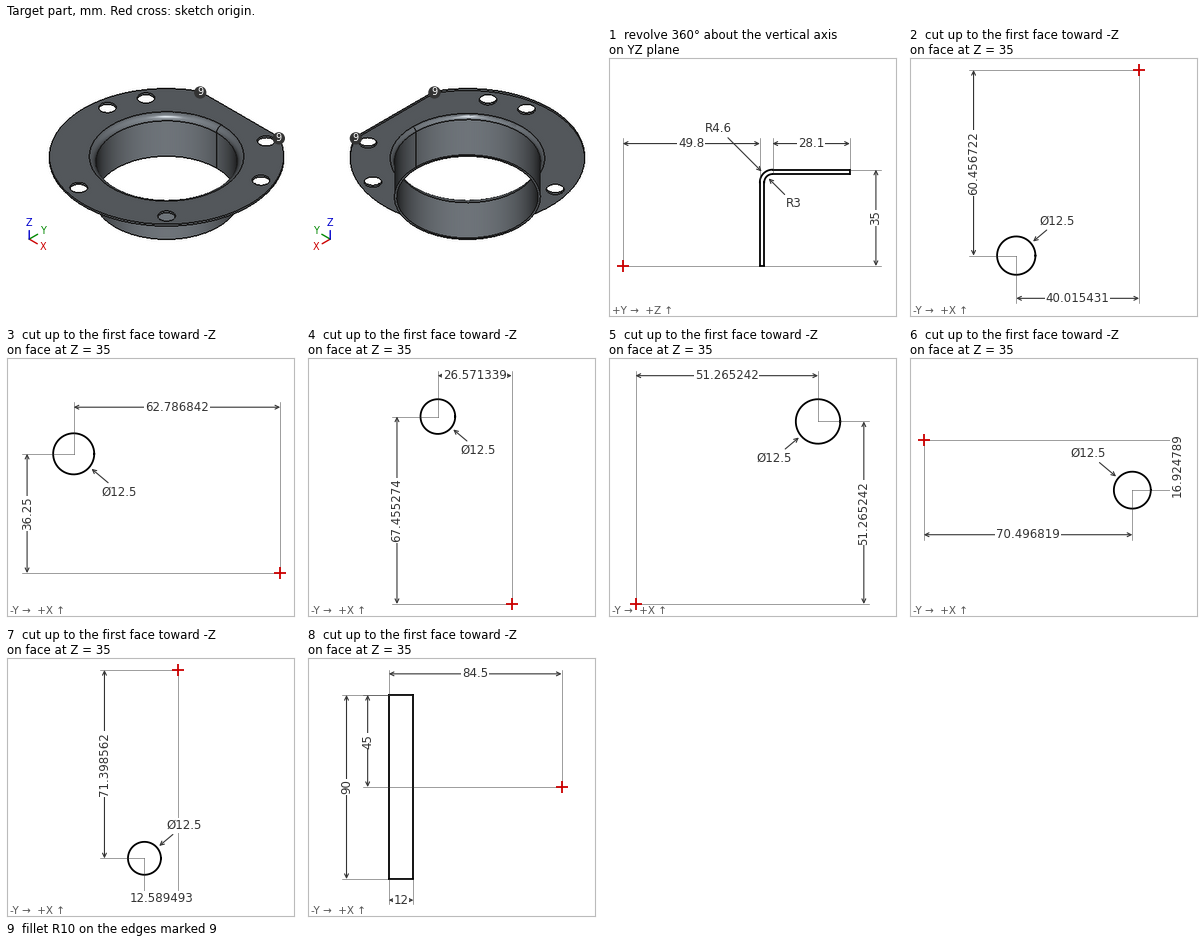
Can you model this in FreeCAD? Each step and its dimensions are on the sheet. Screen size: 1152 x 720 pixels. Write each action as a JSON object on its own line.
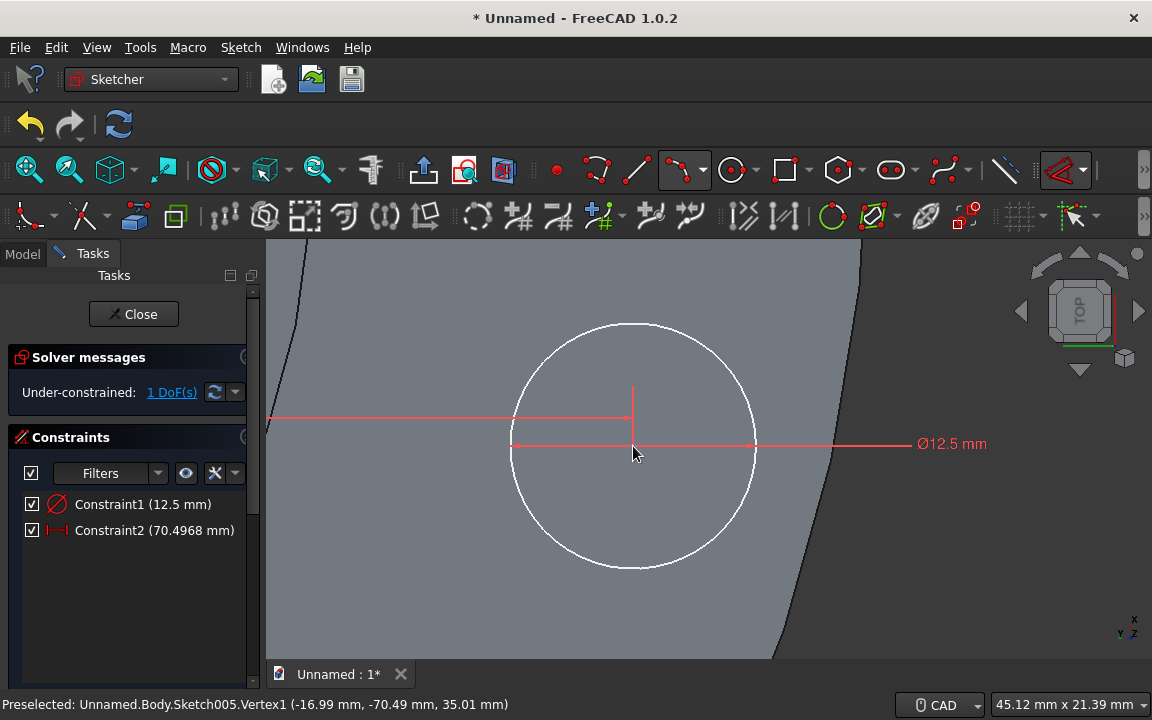
{"action": "left_click", "coordinate": [633, 446]}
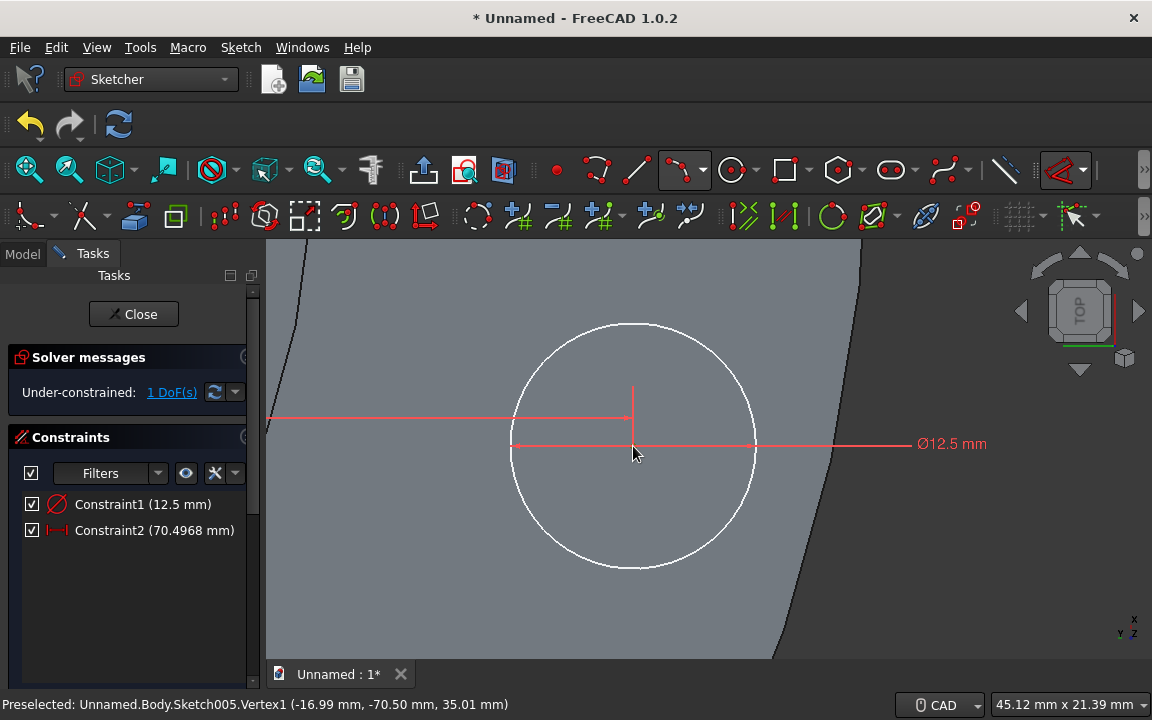
{"action": "key", "text": "i"}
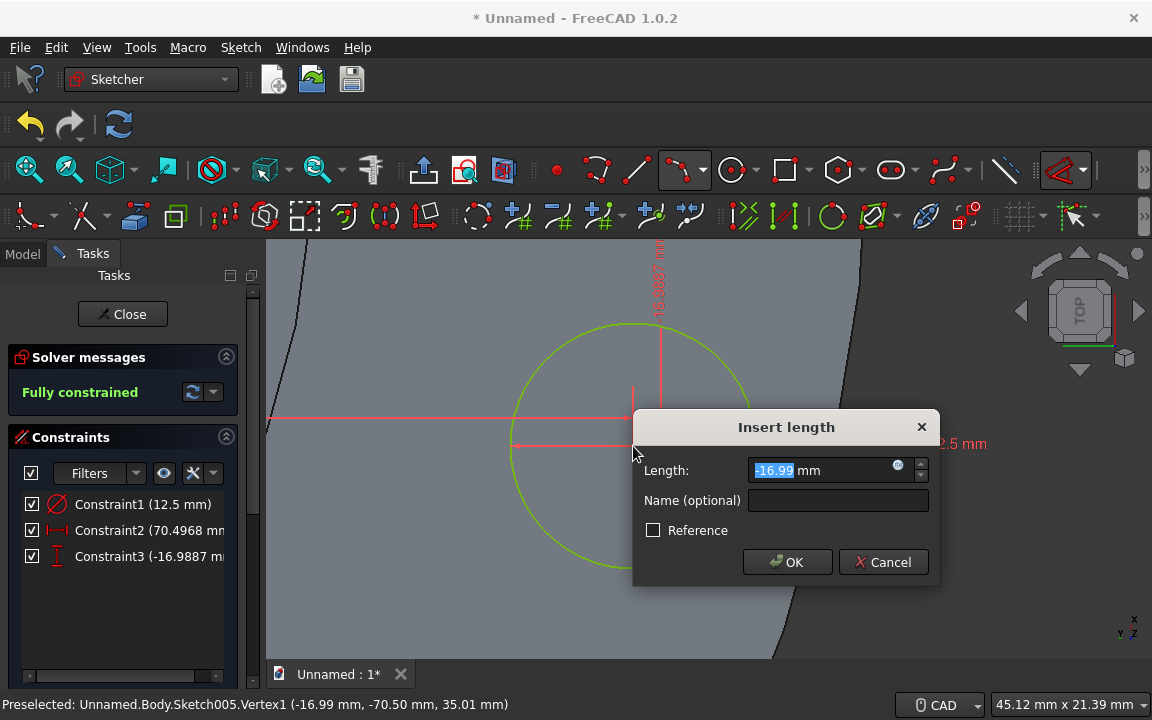
{"action": "type", "text": "-16.924789"}
{"action": "key", "text": "Return"}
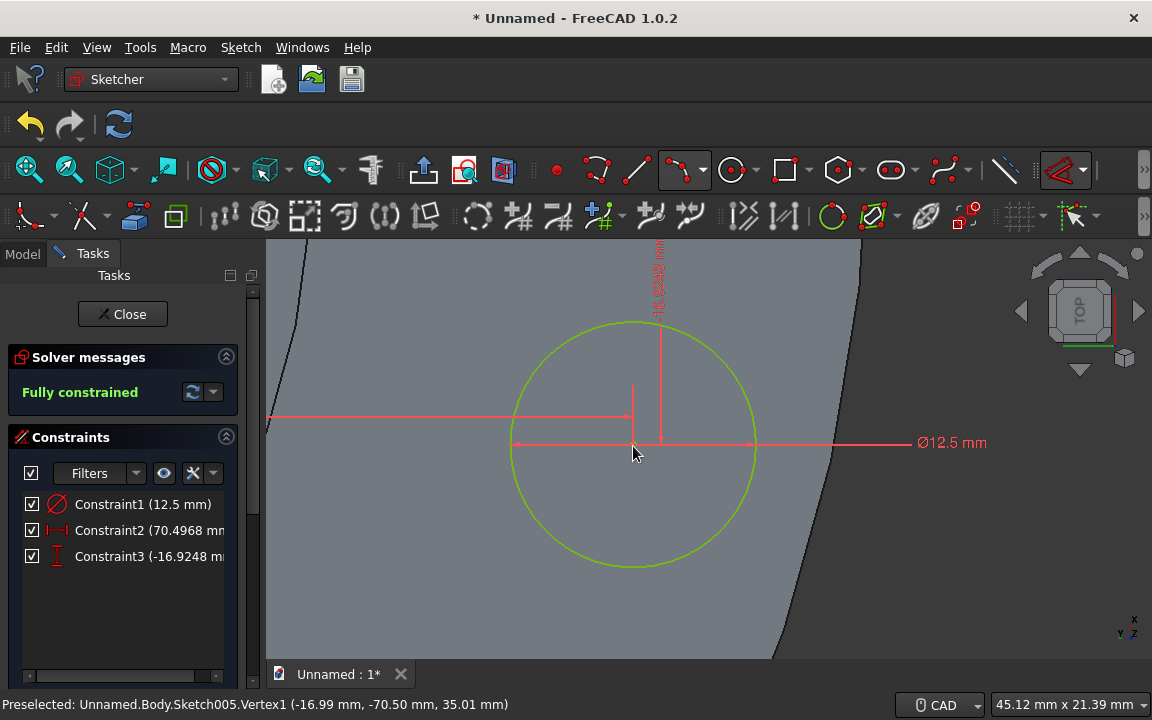
{"action": "left_click", "coordinate": [123, 314]}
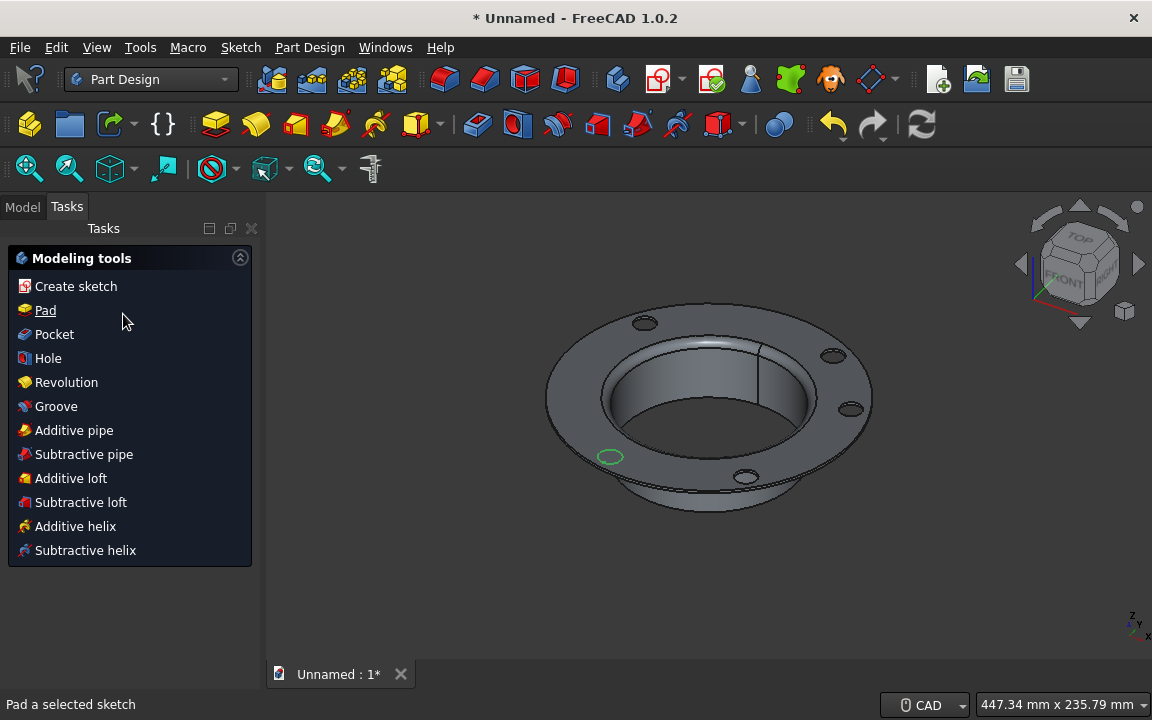
{"action": "left_click", "coordinate": [478, 124]}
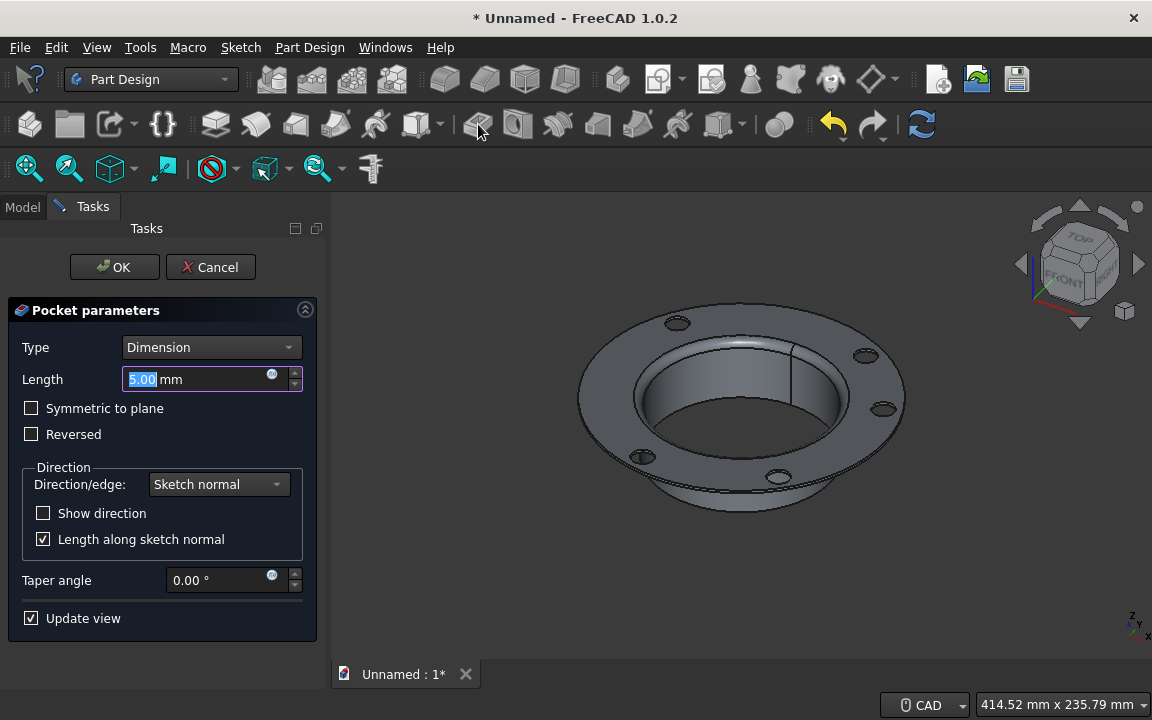
{"action": "left_click", "coordinate": [212, 348]}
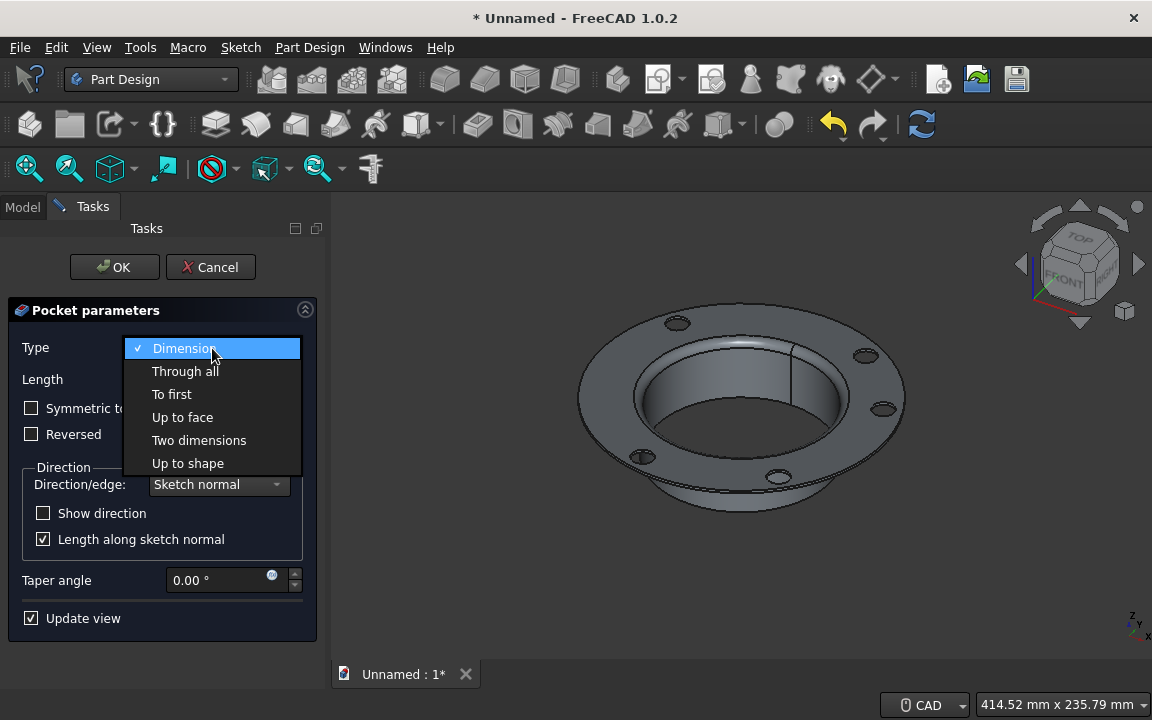
{"action": "left_click", "coordinate": [212, 394]}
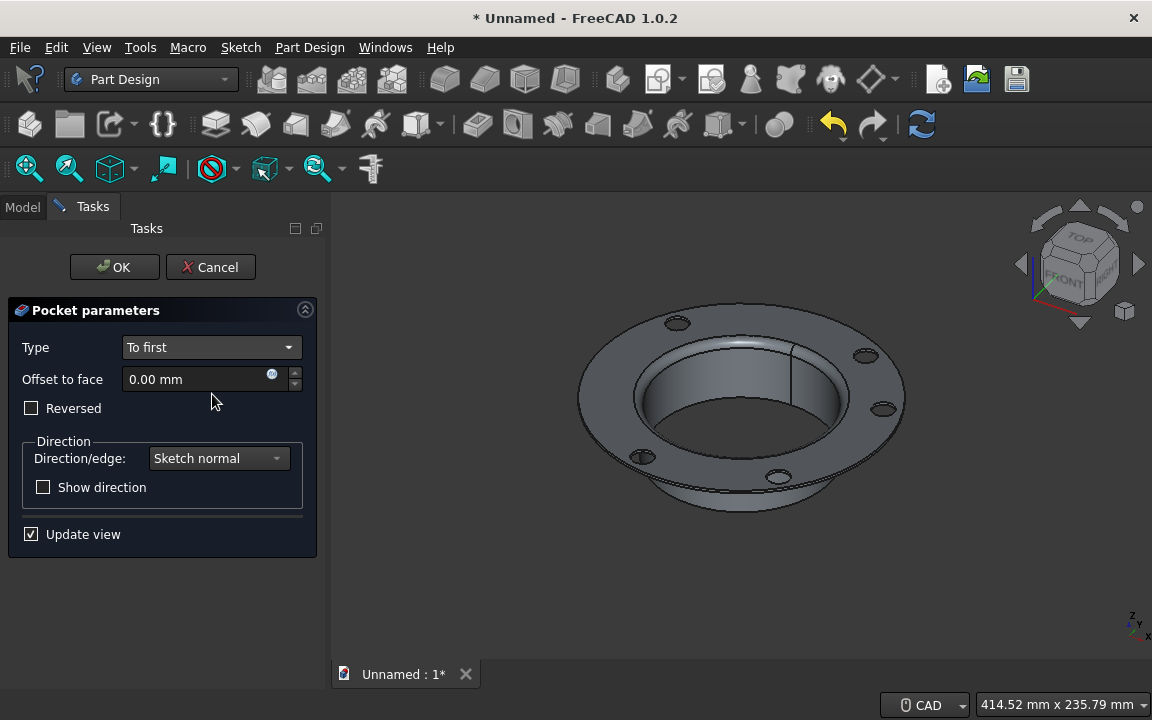
{"action": "left_click", "coordinate": [115, 267]}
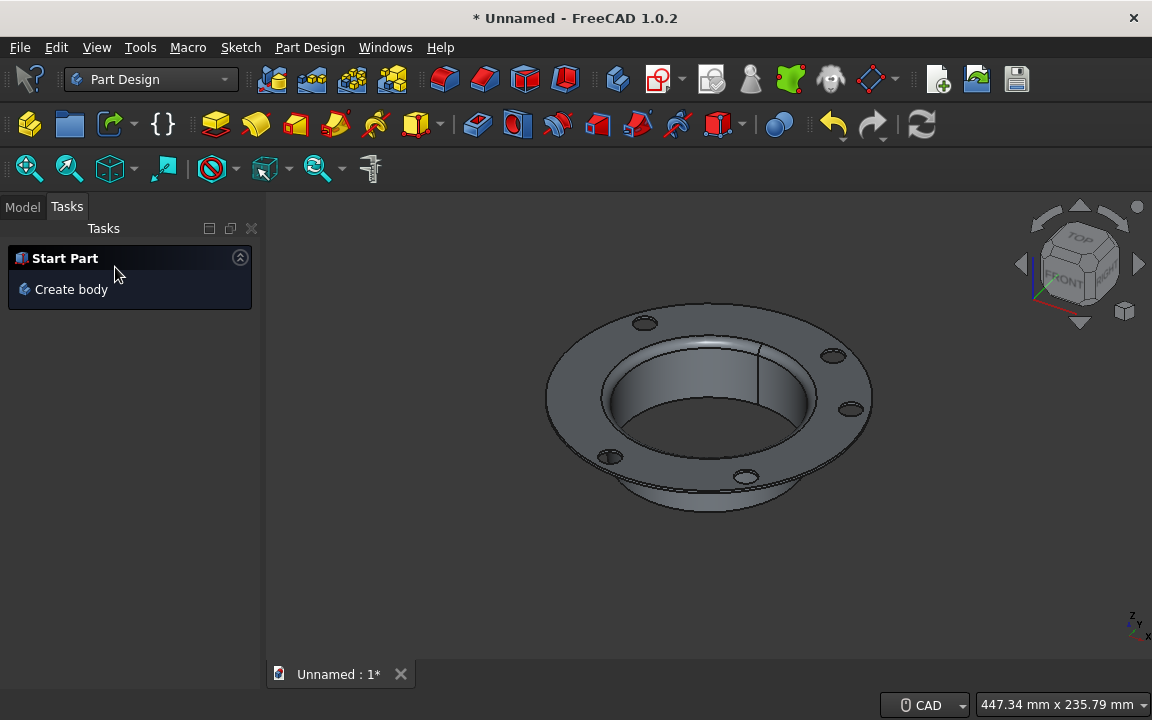
{"action": "left_click", "coordinate": [837, 377]}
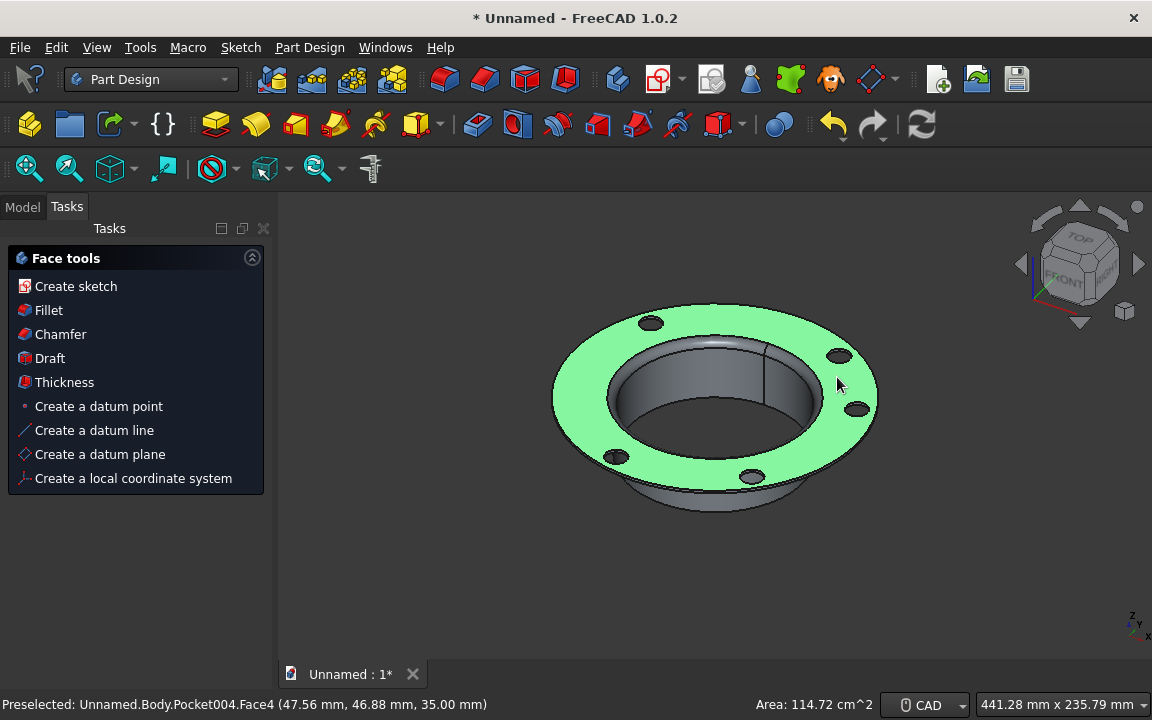
{"action": "left_click", "coordinate": [658, 80]}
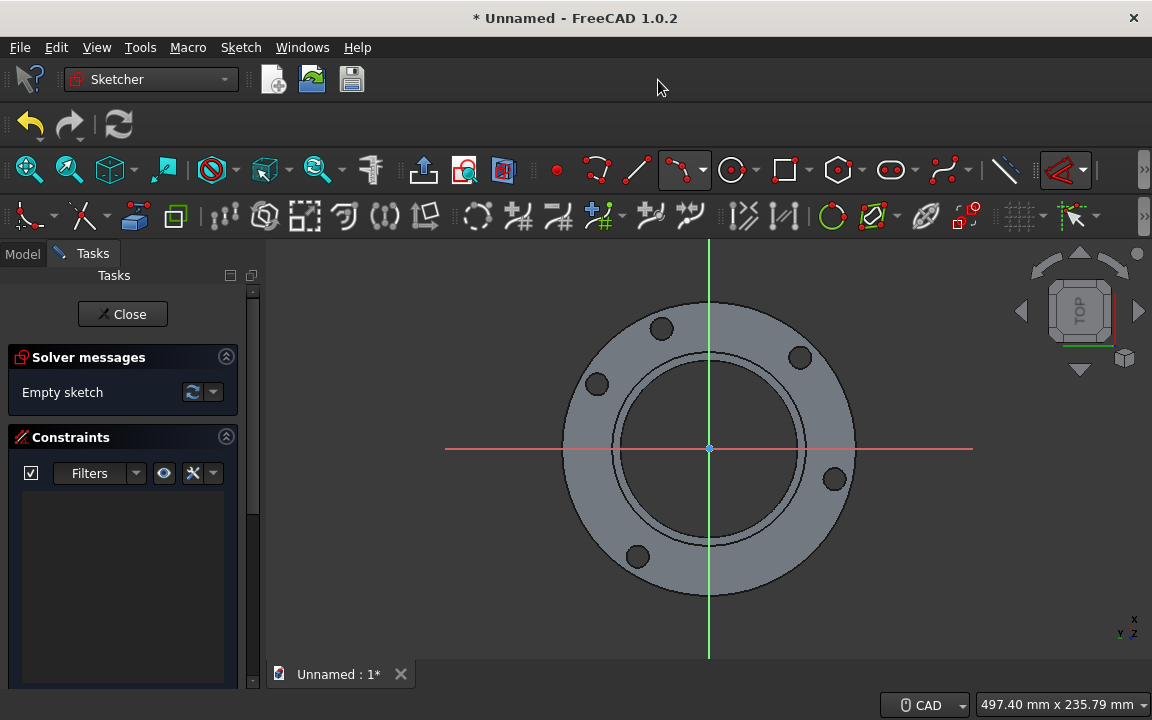
{"action": "scroll", "coordinate": [691, 589], "scroll_direction": "up", "scroll_amount": 12}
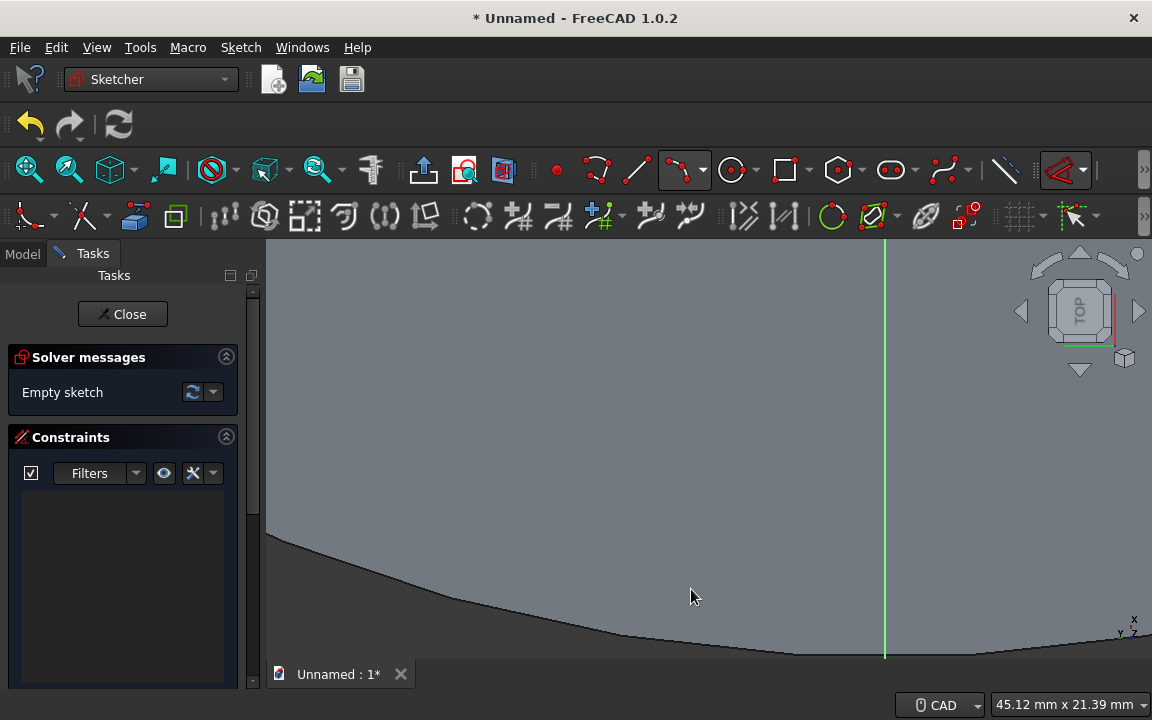
{"action": "key", "text": "g c"}